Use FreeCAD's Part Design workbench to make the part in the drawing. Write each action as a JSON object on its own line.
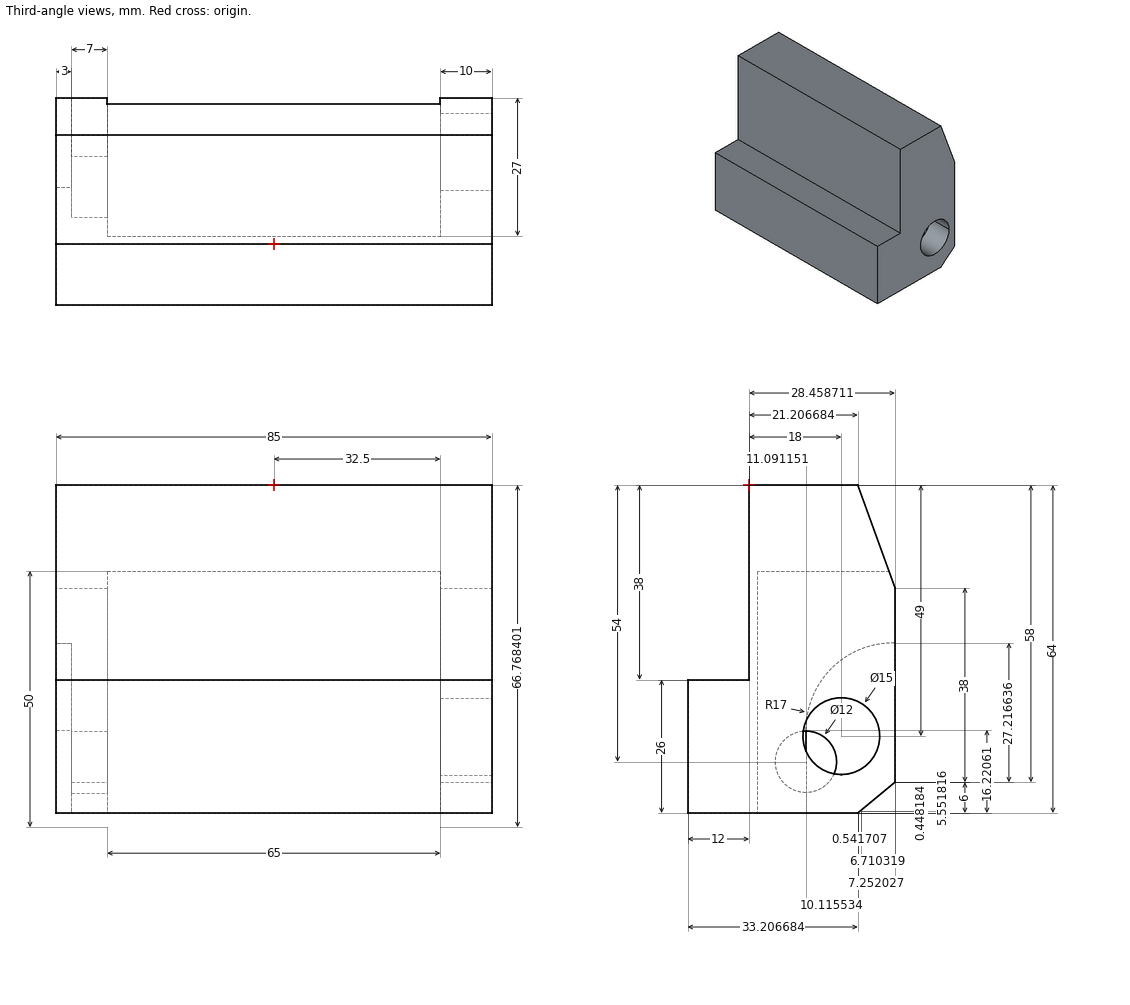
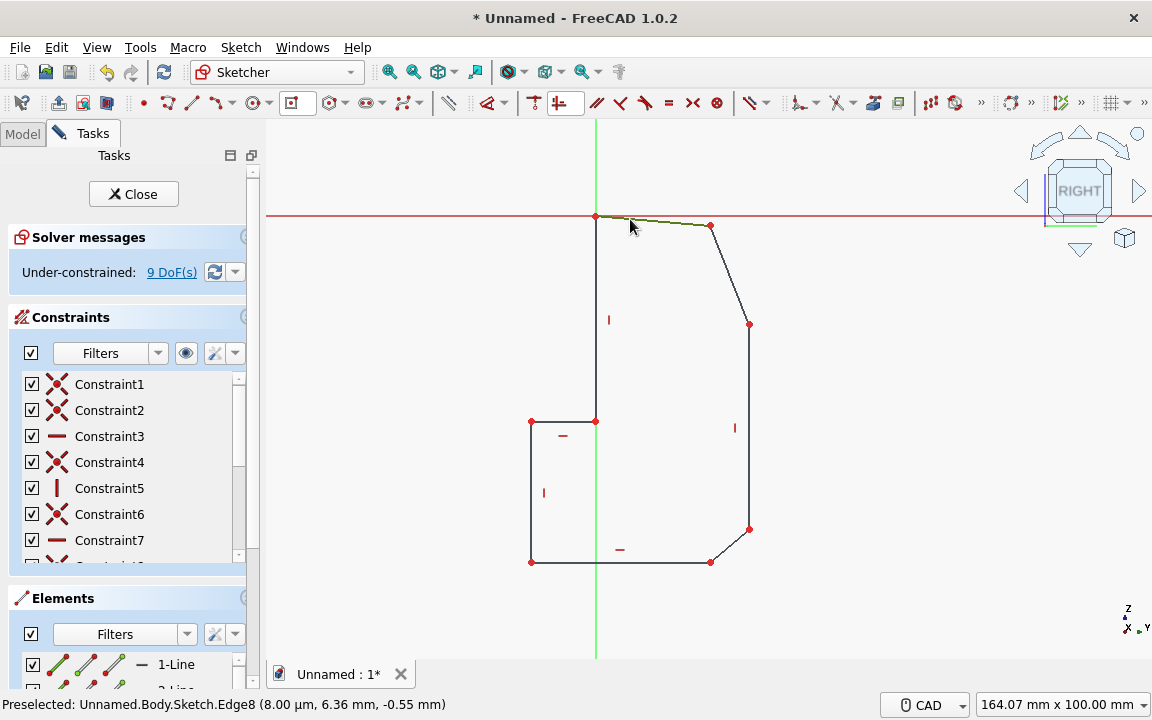
{"action": "left_click", "coordinate": [578, 104]}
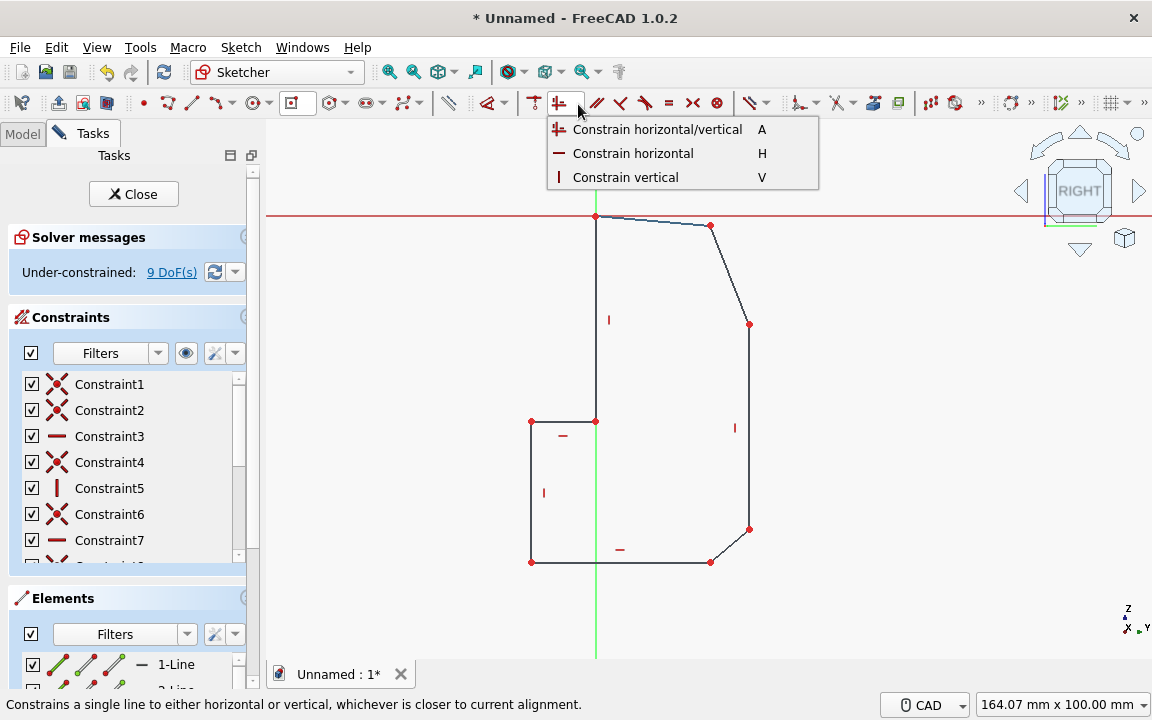
{"action": "left_click", "coordinate": [683, 153]}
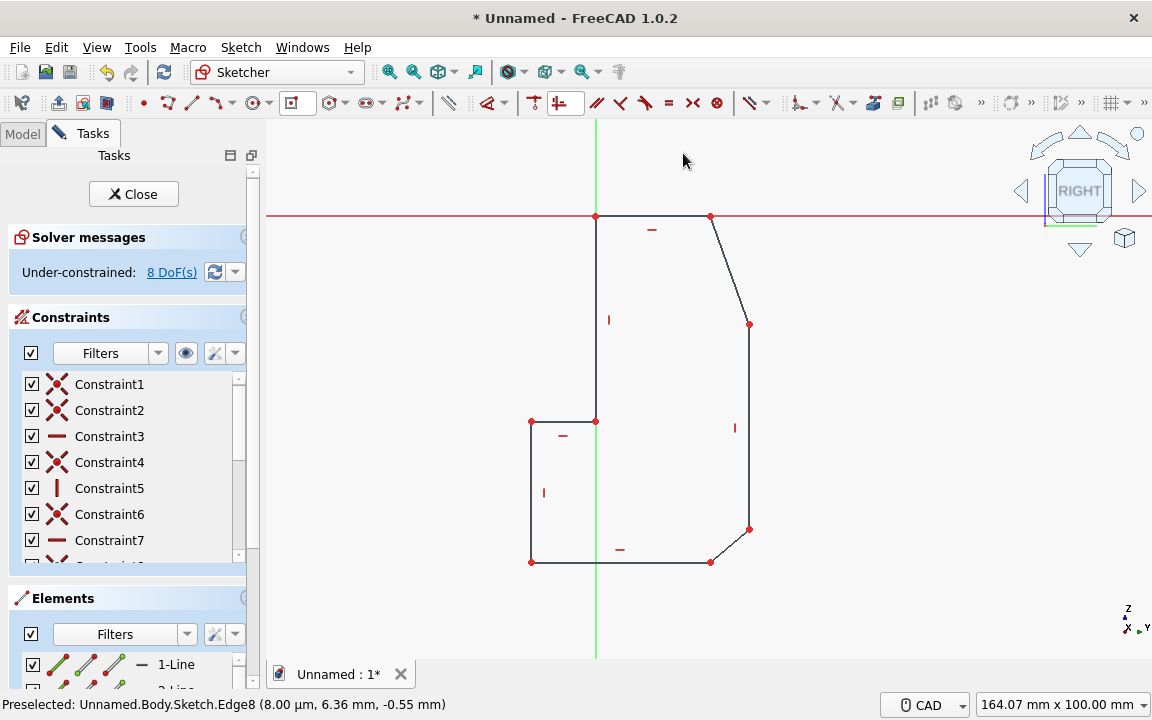
{"action": "left_click", "coordinate": [488, 104]}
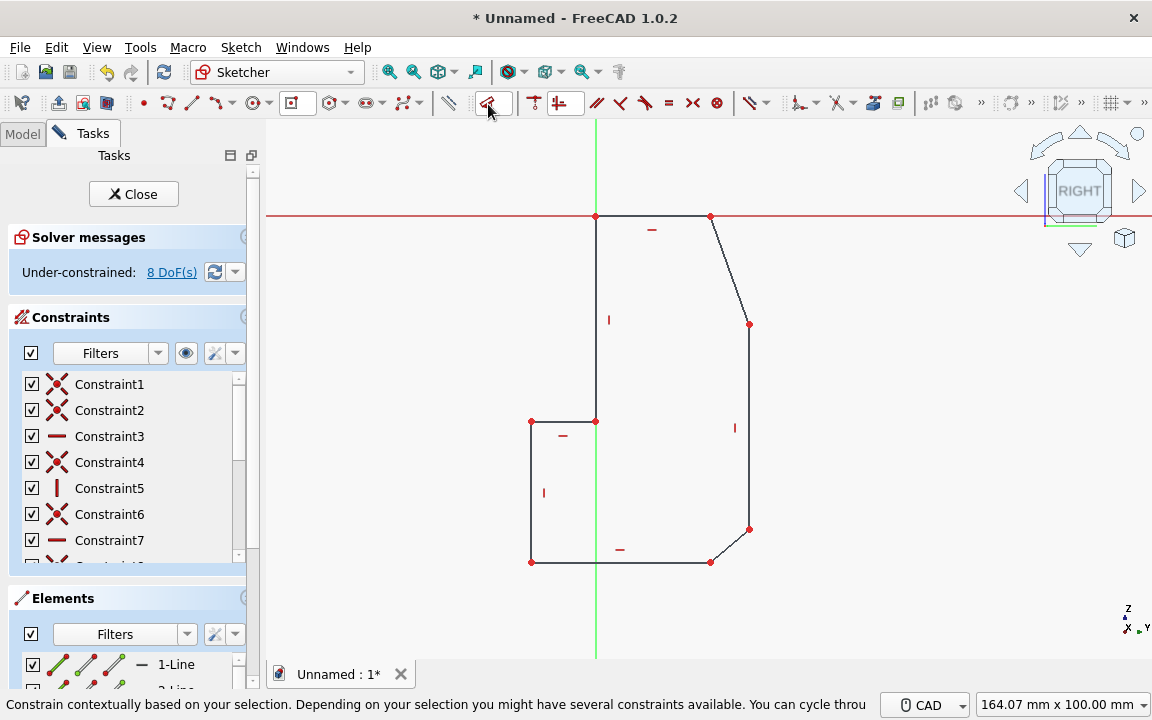
{"action": "left_click", "coordinate": [596, 278]}
{"action": "left_click", "coordinate": [562, 319]}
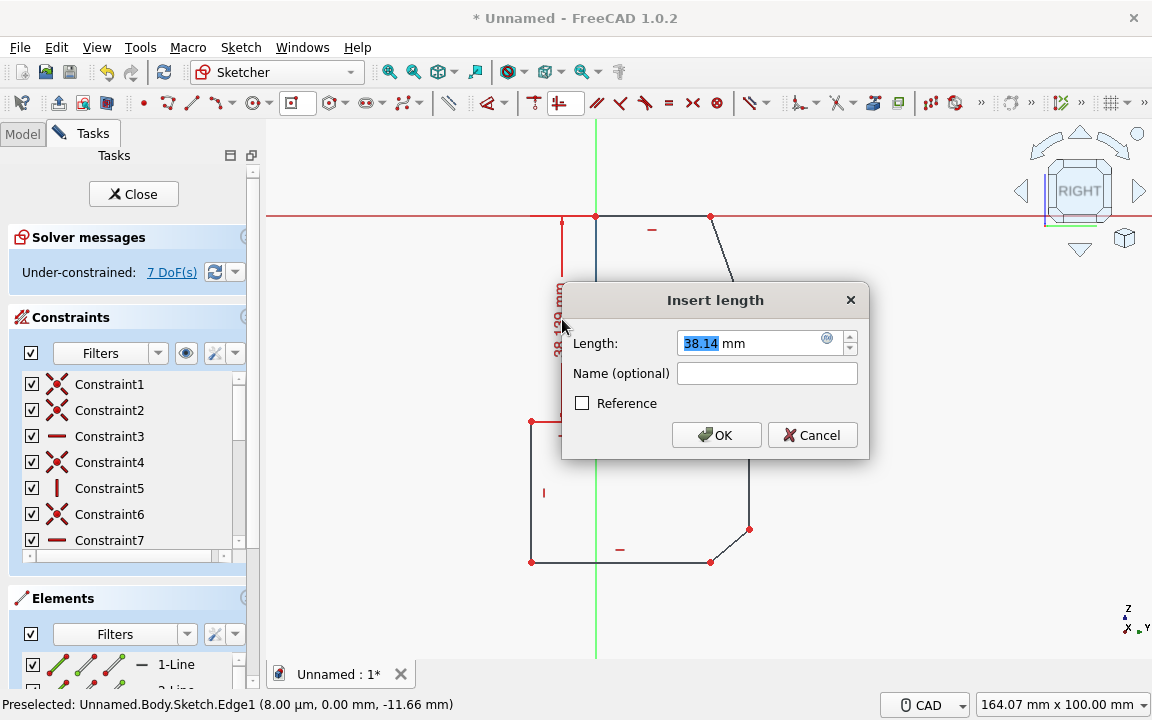
{"action": "type", "text": "38"}
{"action": "key", "text": "Return"}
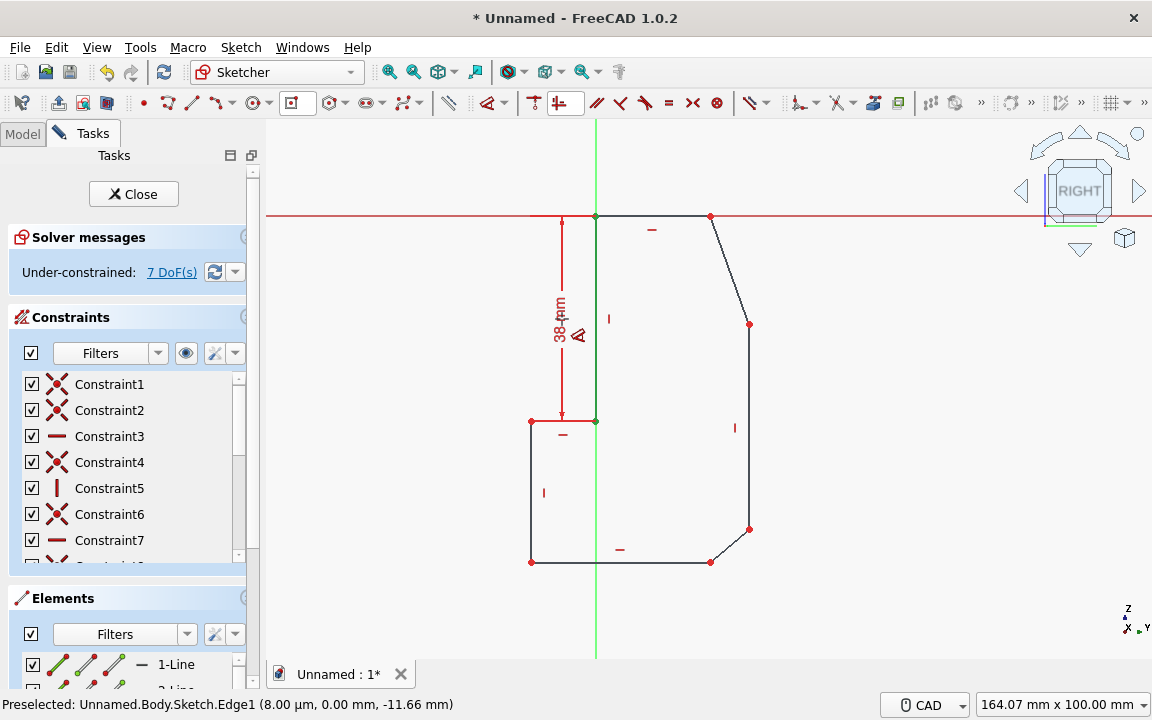
{"action": "left_click", "coordinate": [576, 421]}
{"action": "left_click", "coordinate": [563, 455]}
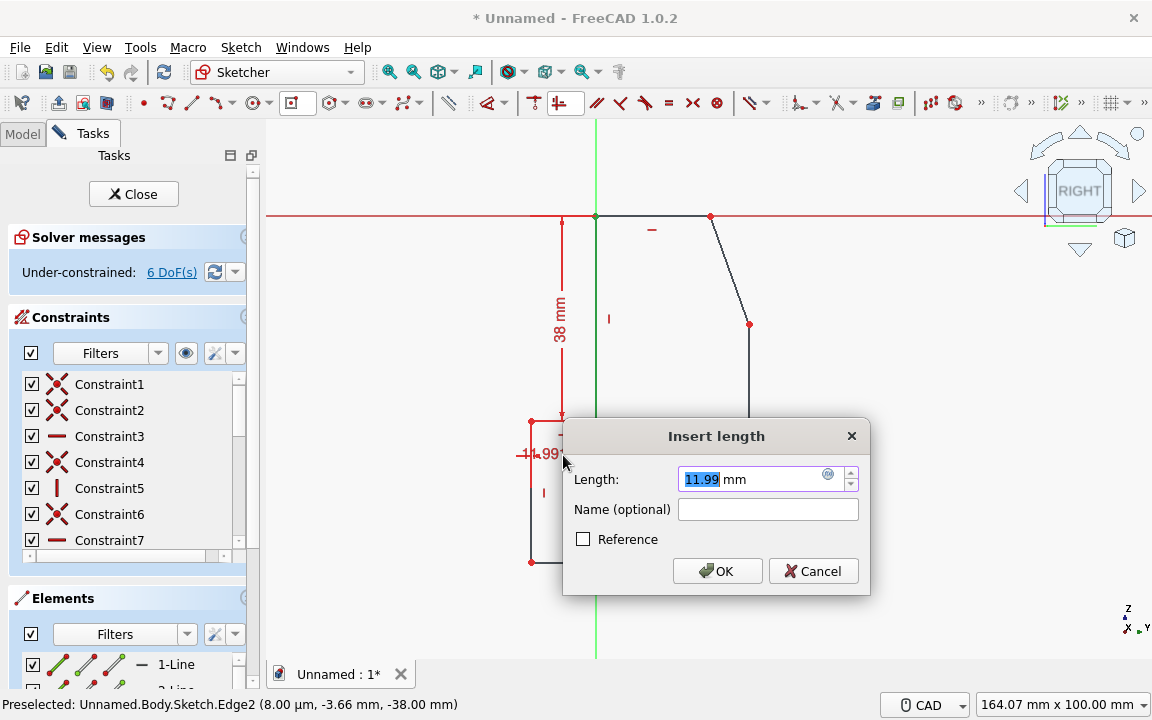
{"action": "type", "text": "12"}
{"action": "key", "text": "Return"}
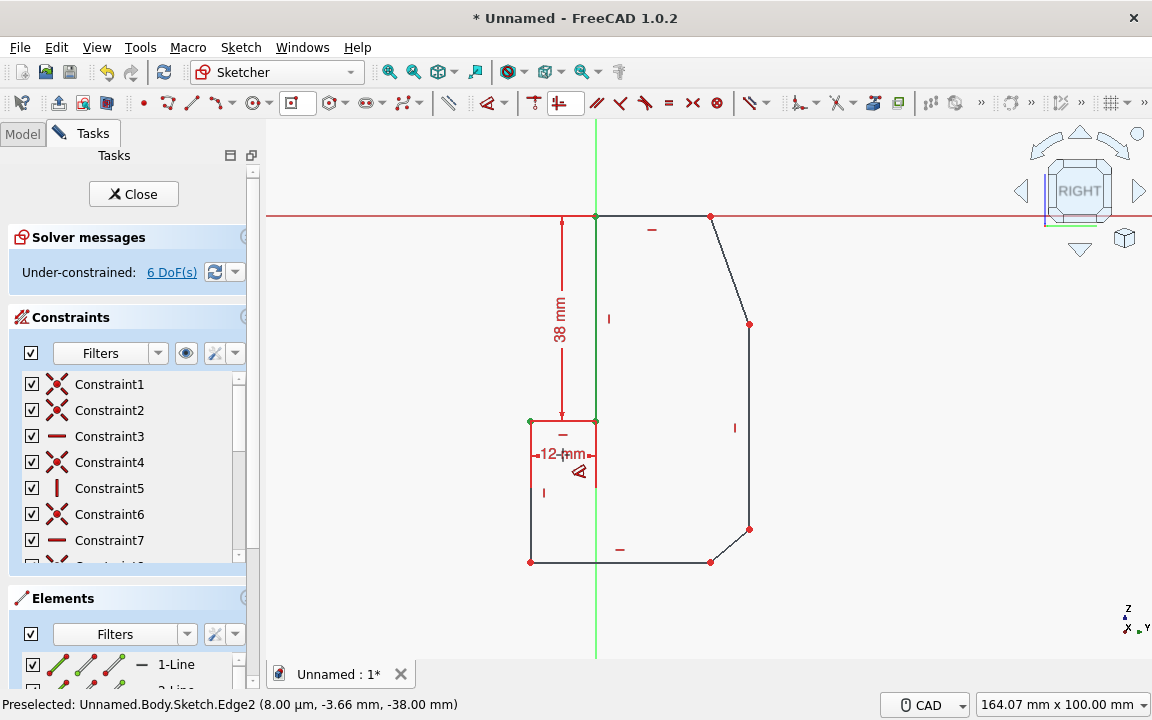
{"action": "left_click", "coordinate": [531, 464]}
{"action": "left_click", "coordinate": [497, 492]}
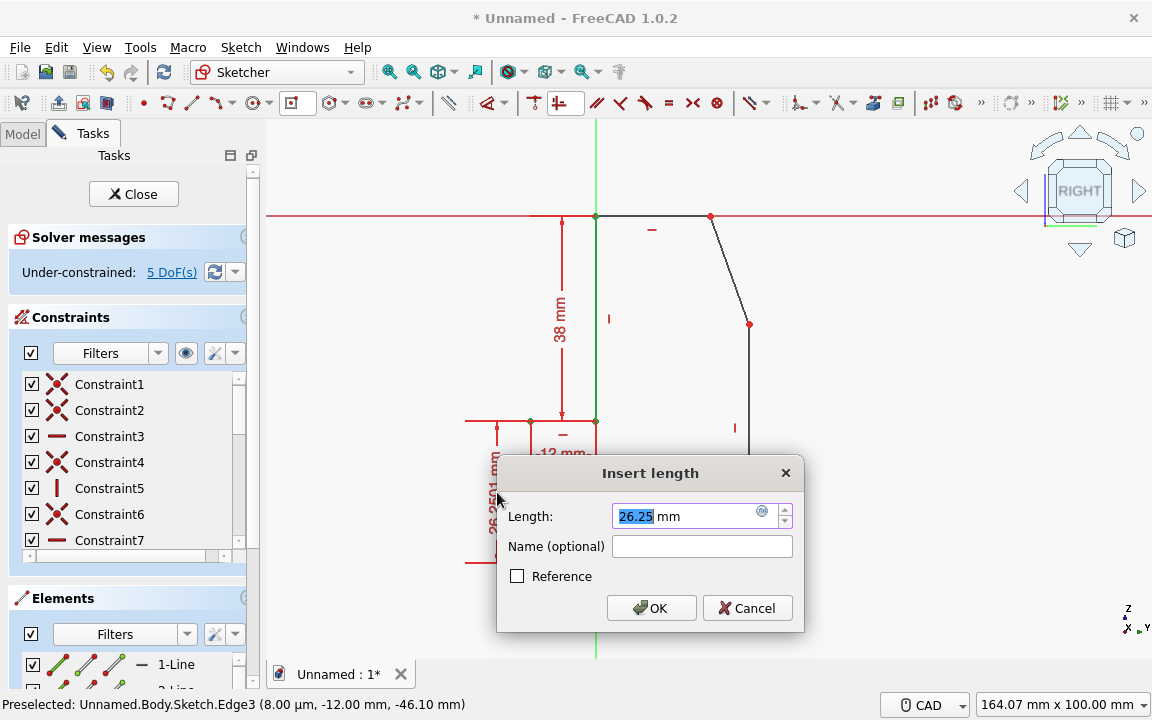
{"action": "type", "text": "26"}
{"action": "key", "text": "Return"}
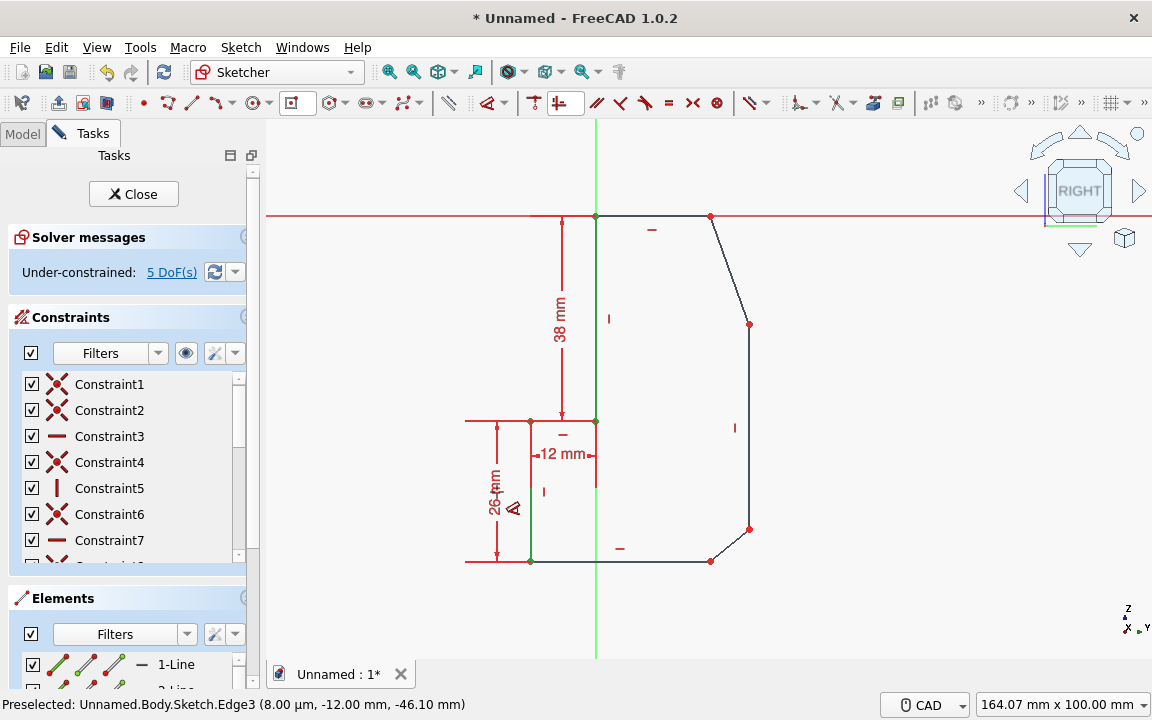
{"action": "left_click", "coordinate": [749, 468]}
{"action": "left_click", "coordinate": [783, 427]}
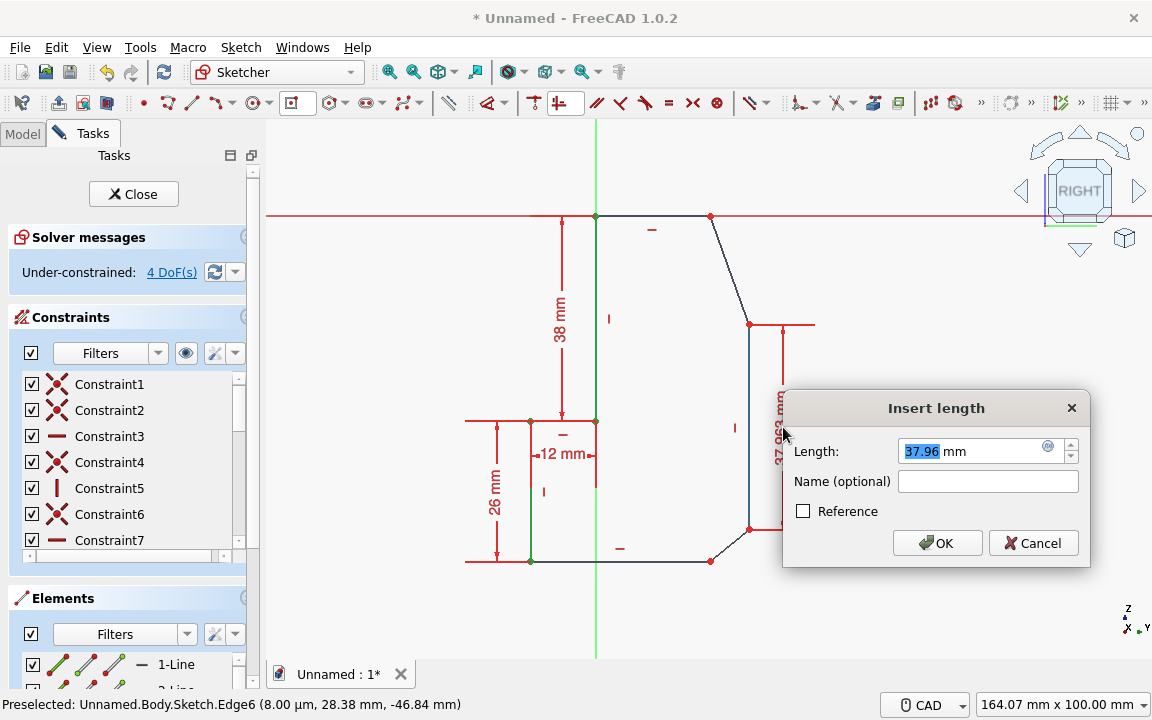
{"action": "type", "text": "38"}
{"action": "key", "text": "Return"}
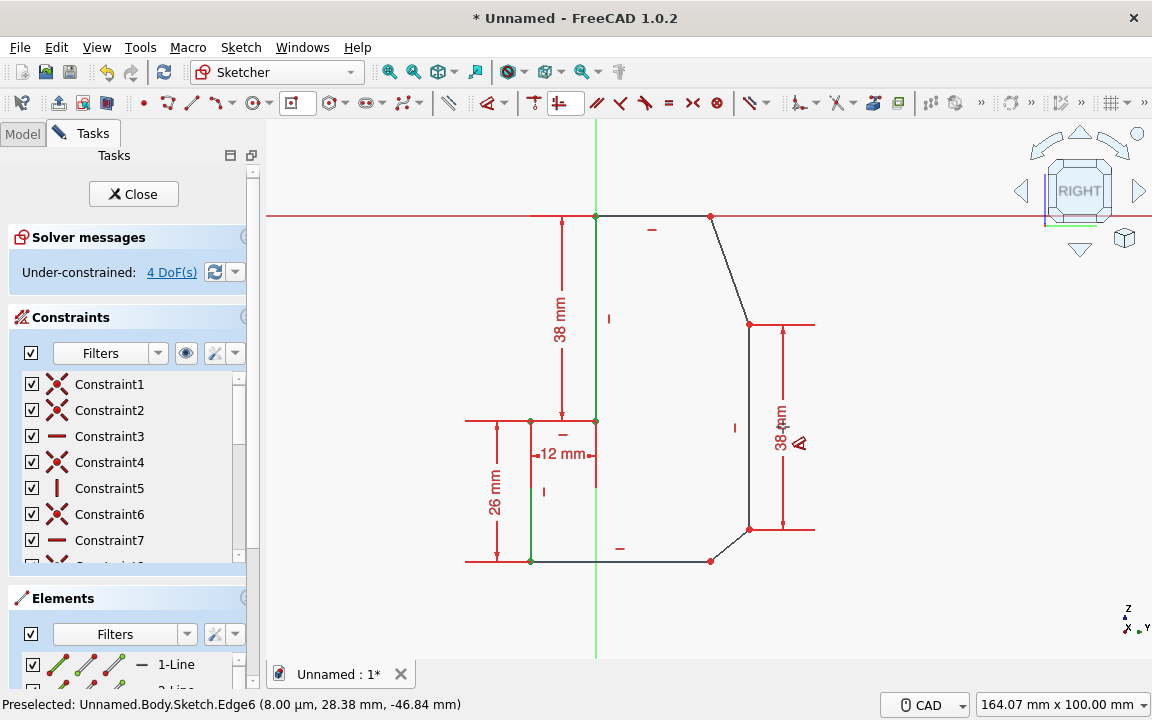
{"action": "scroll", "coordinate": [722, 552], "scroll_direction": "up", "scroll_amount": 2}